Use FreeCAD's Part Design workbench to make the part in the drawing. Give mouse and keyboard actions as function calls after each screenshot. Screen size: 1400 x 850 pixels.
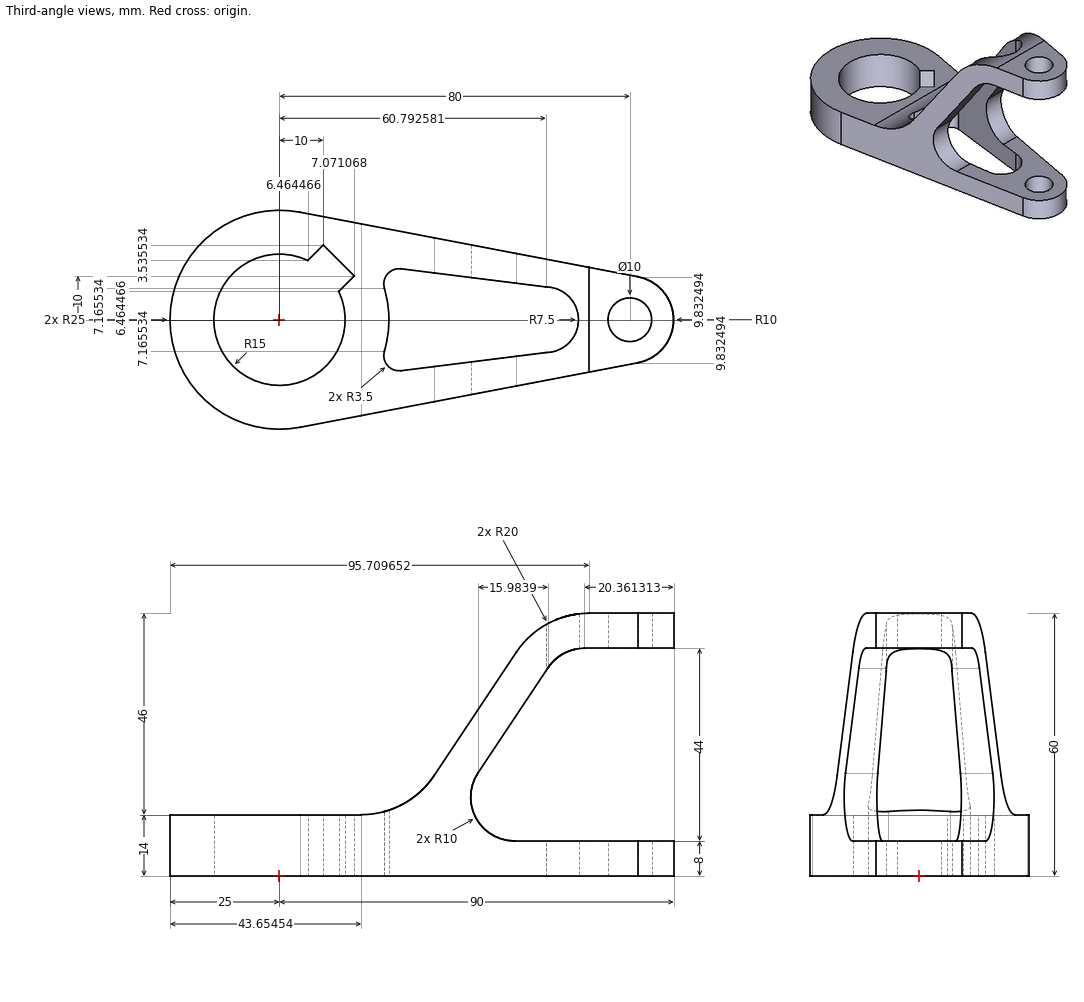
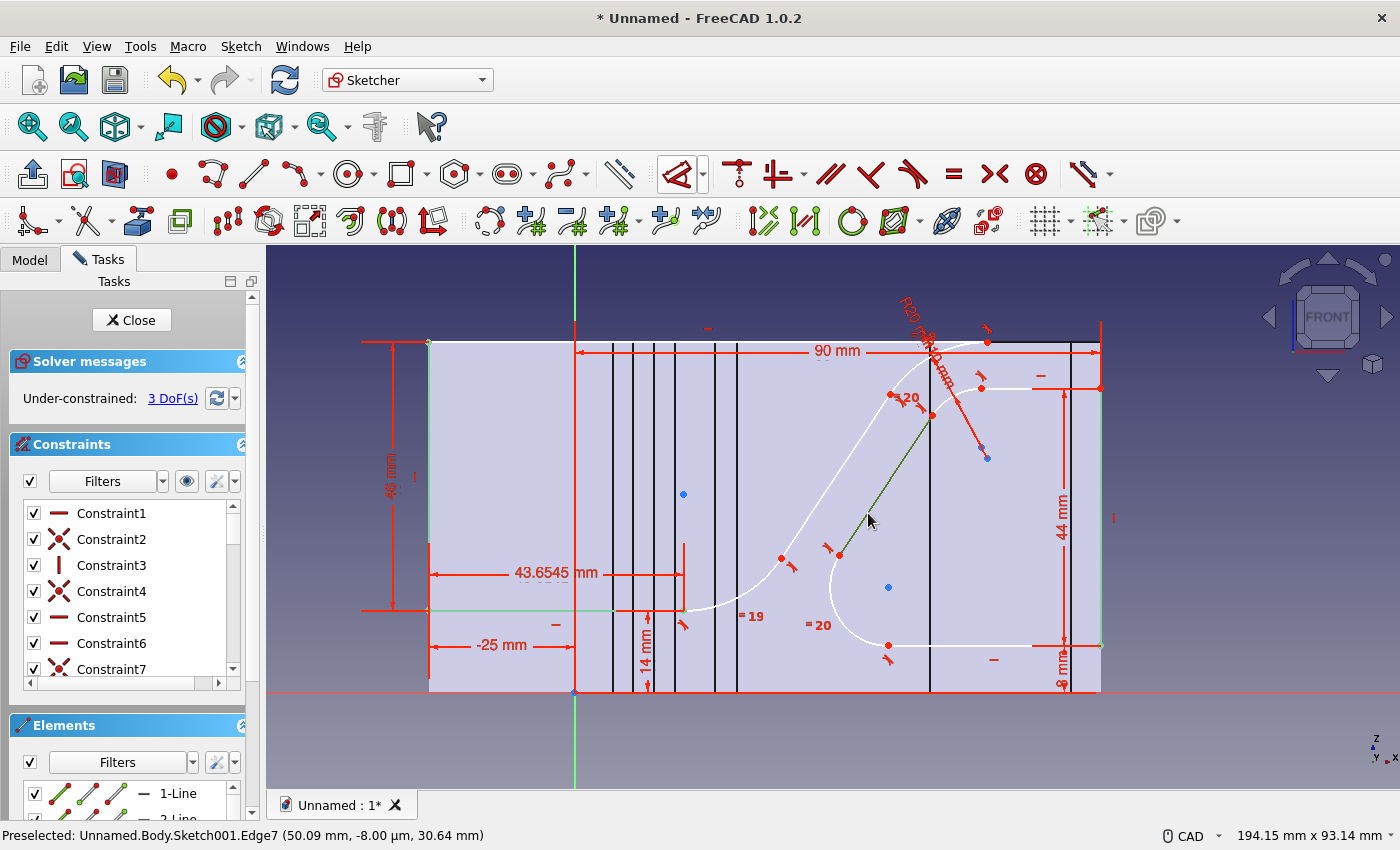
key(l)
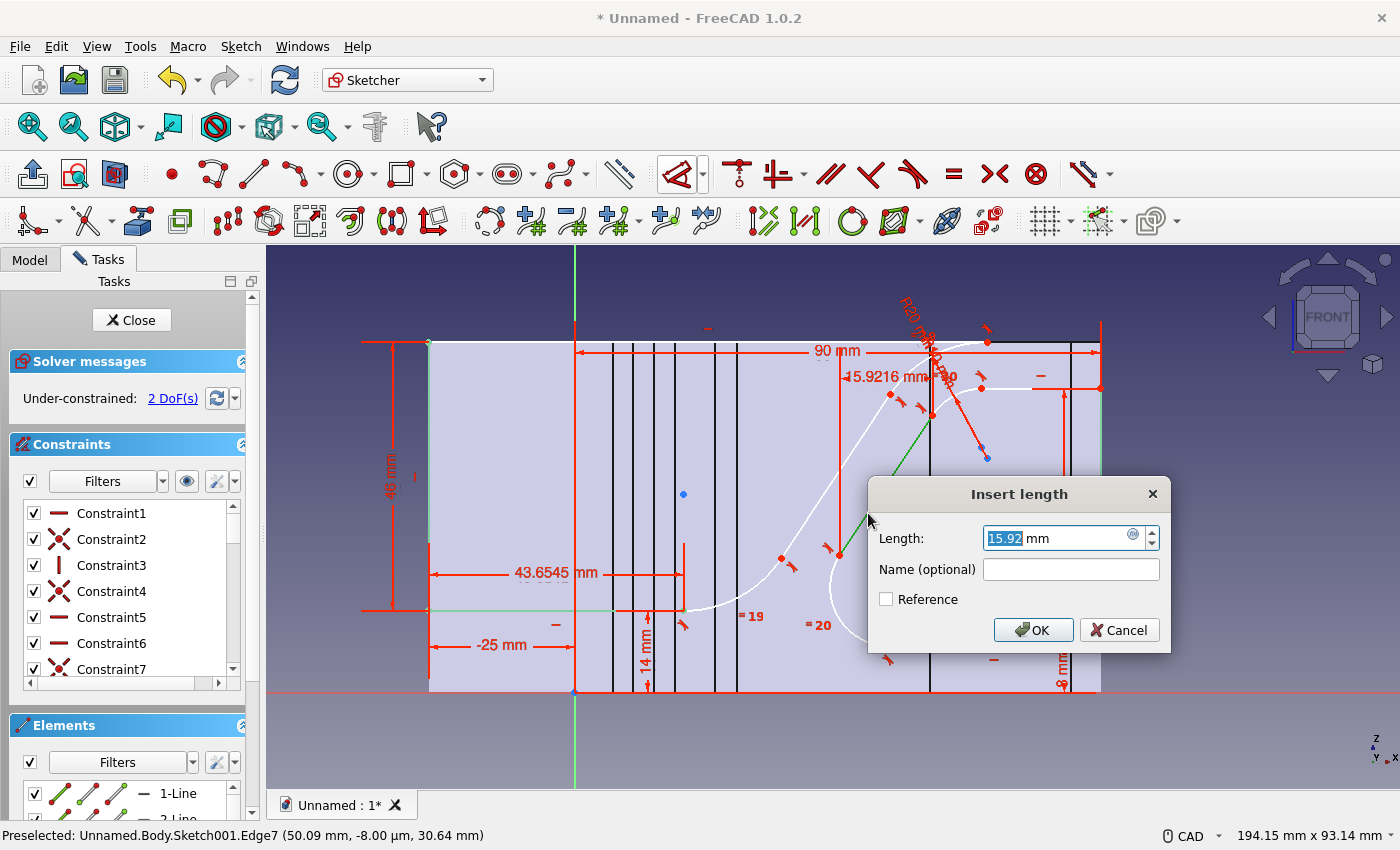
text(15.9839)
key(Return)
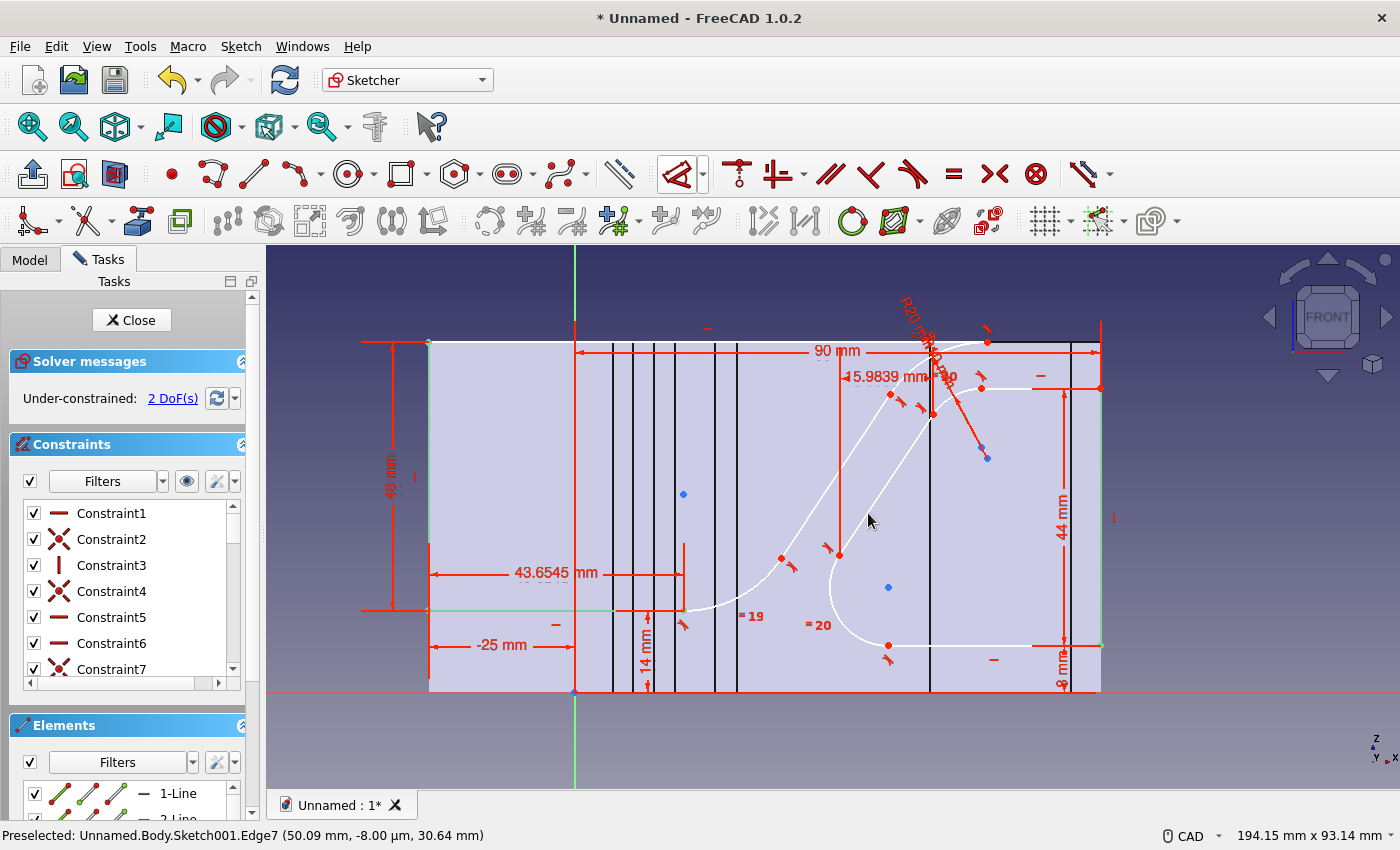
click(596, 342)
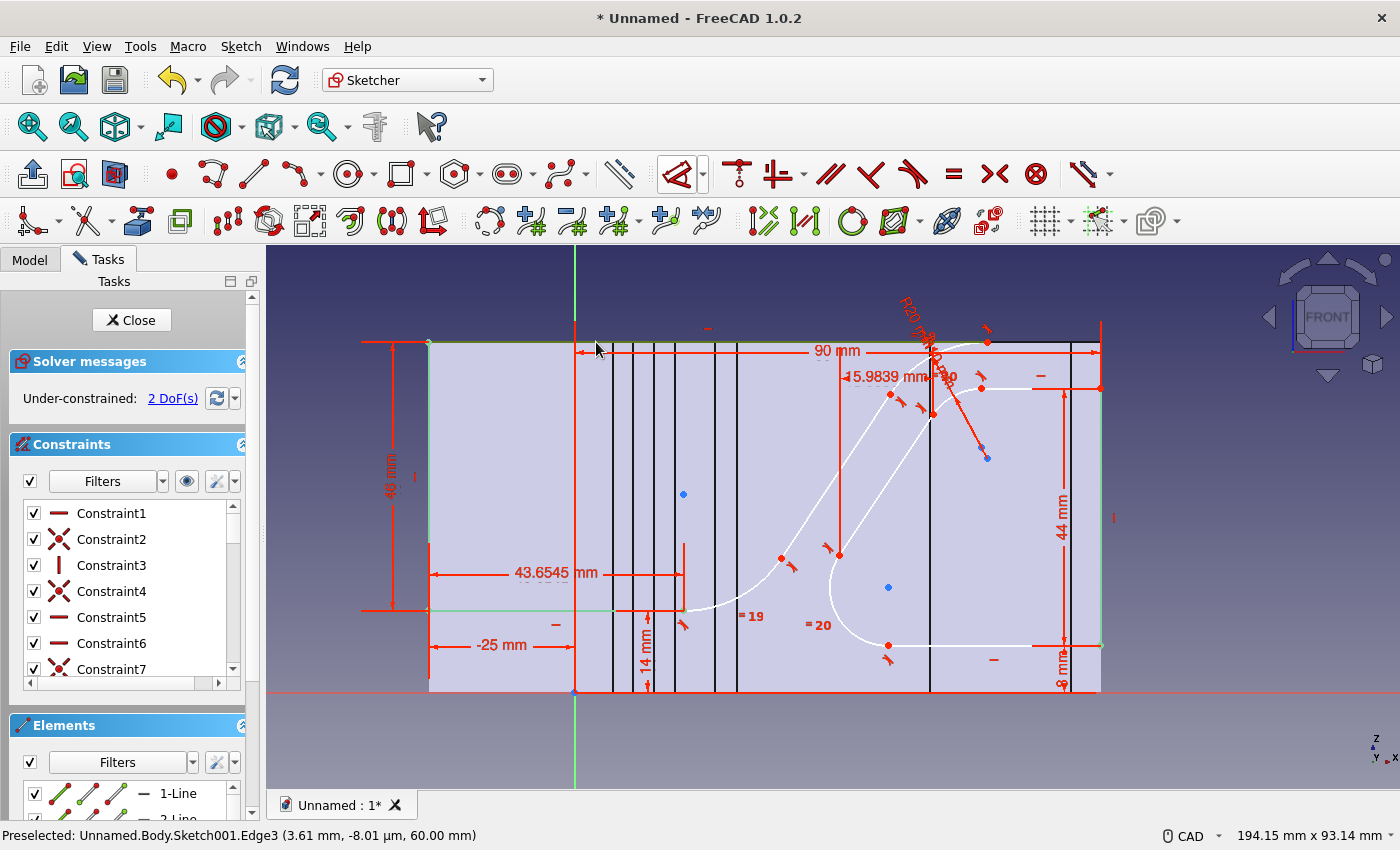
key(l)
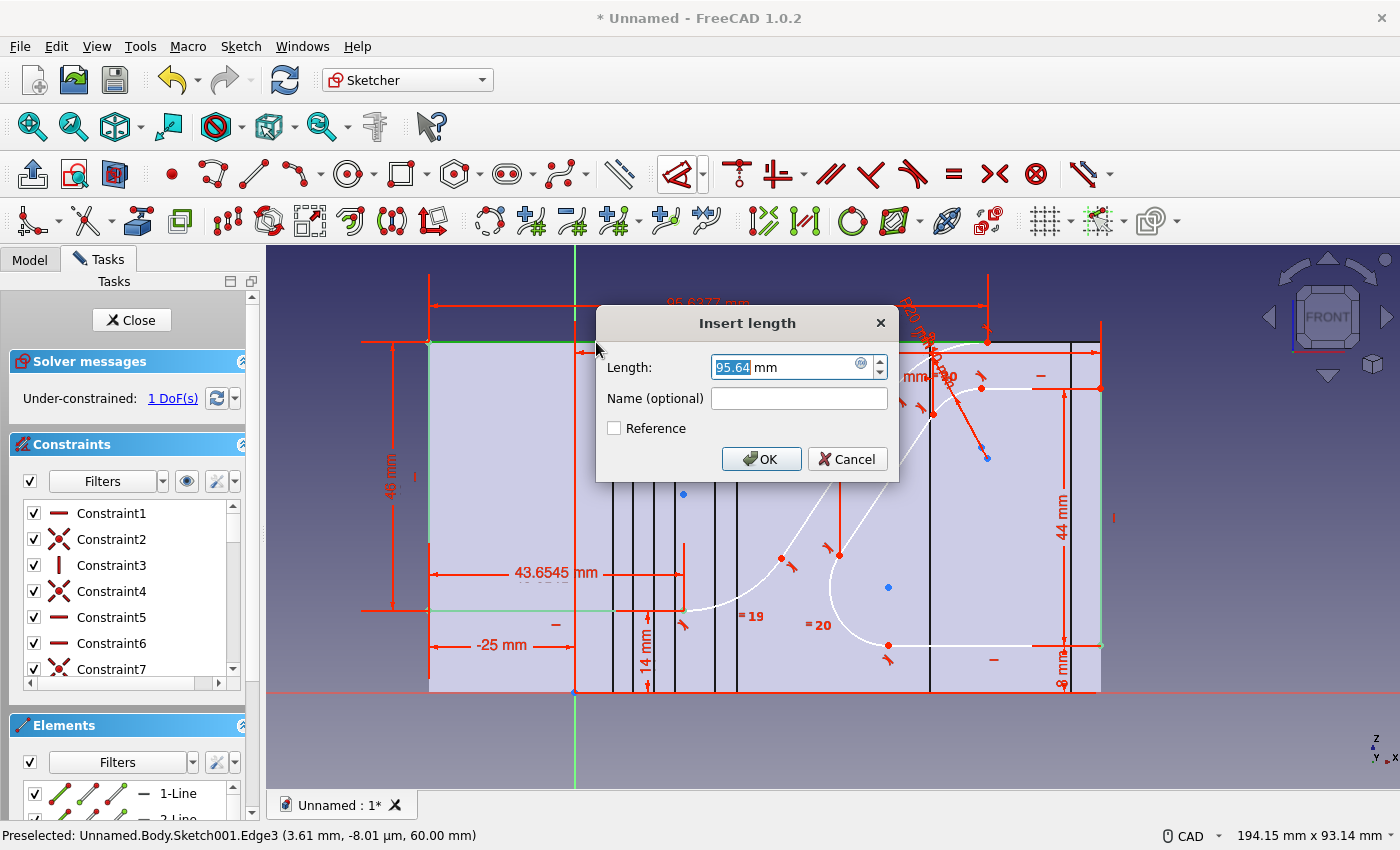
text(95.709652)
key(Return)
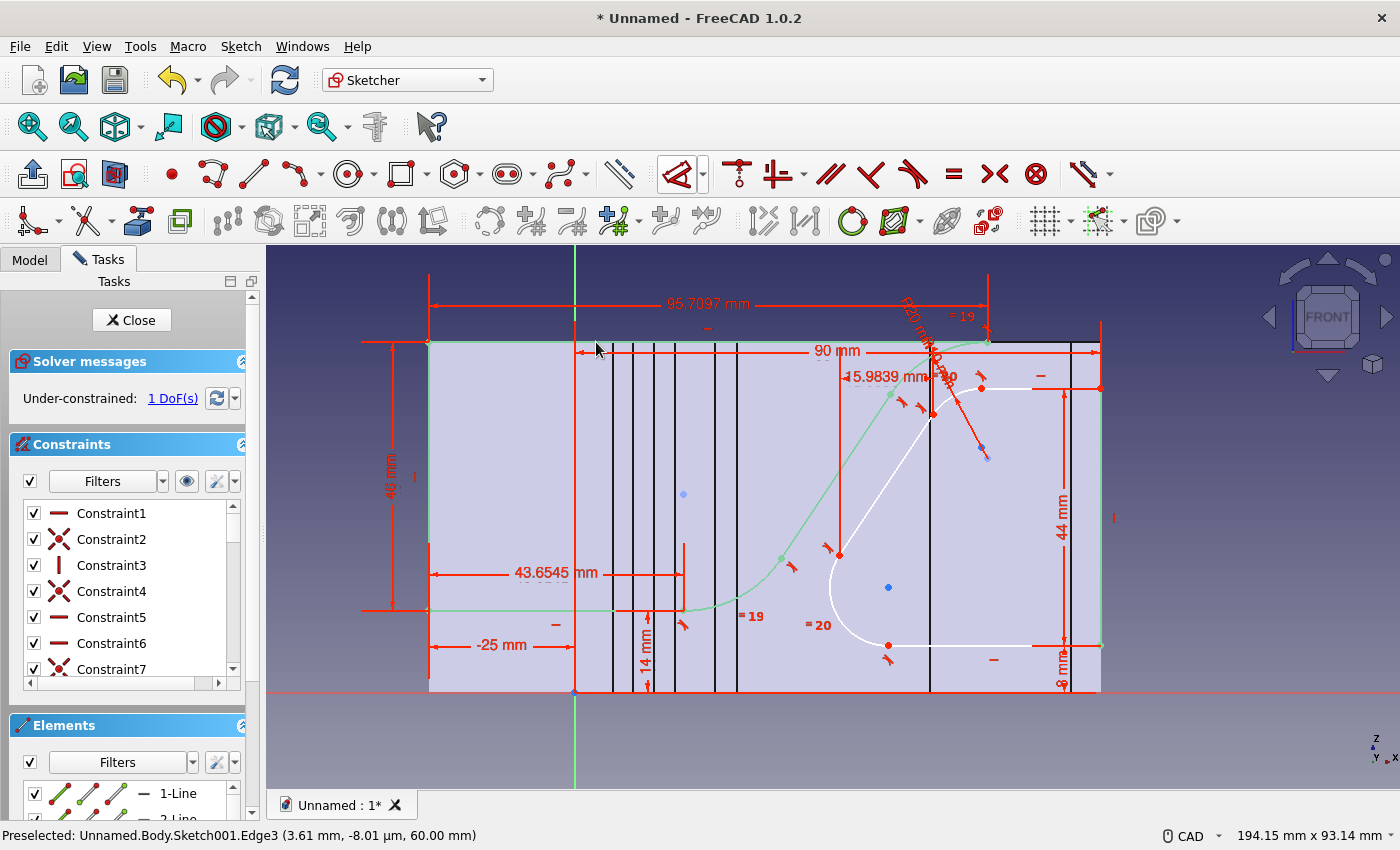
click(1017, 389)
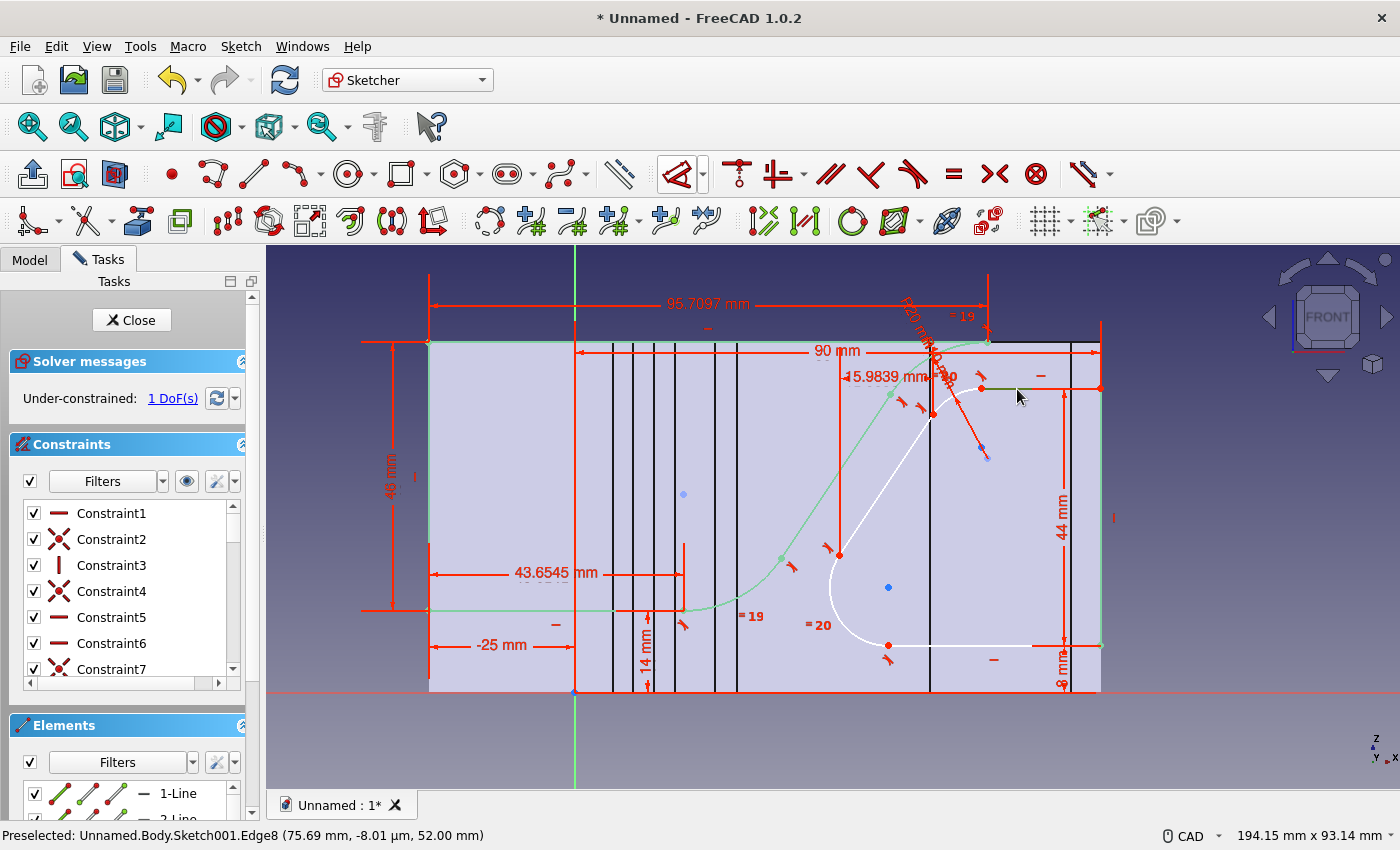
click(702, 174)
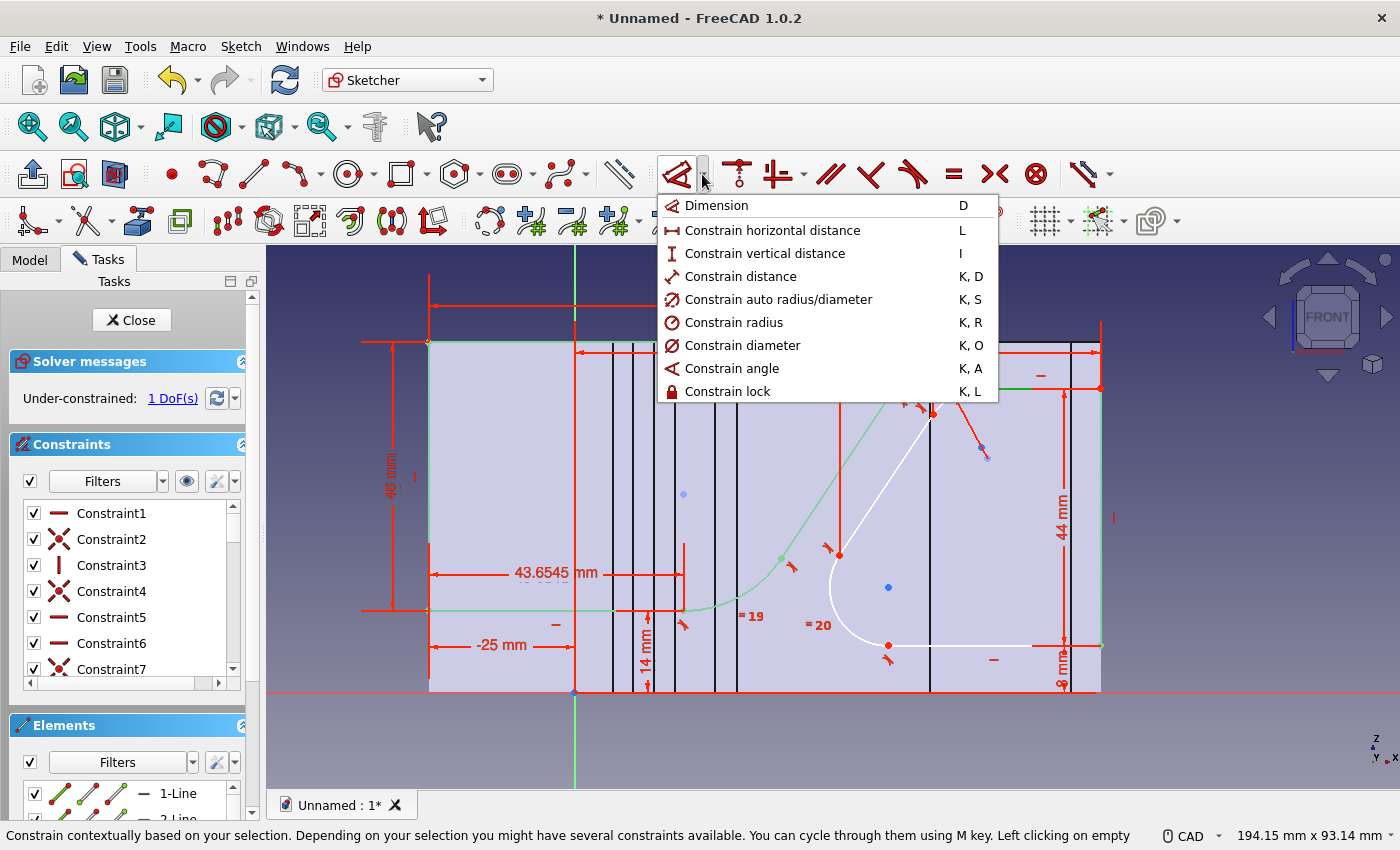
click(828, 230)